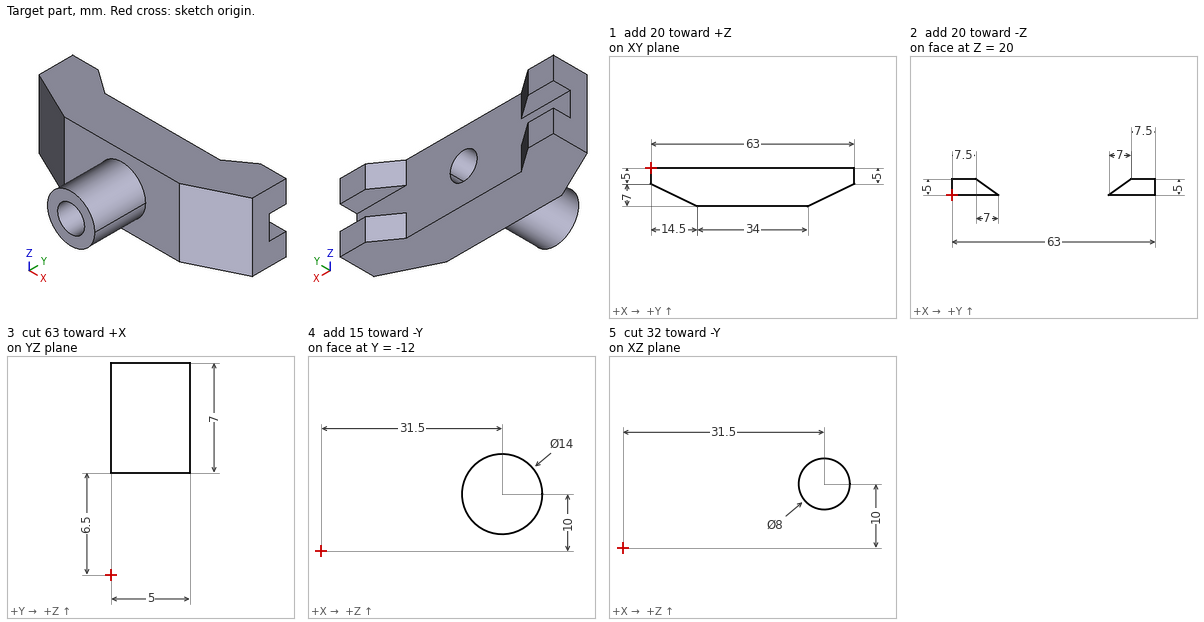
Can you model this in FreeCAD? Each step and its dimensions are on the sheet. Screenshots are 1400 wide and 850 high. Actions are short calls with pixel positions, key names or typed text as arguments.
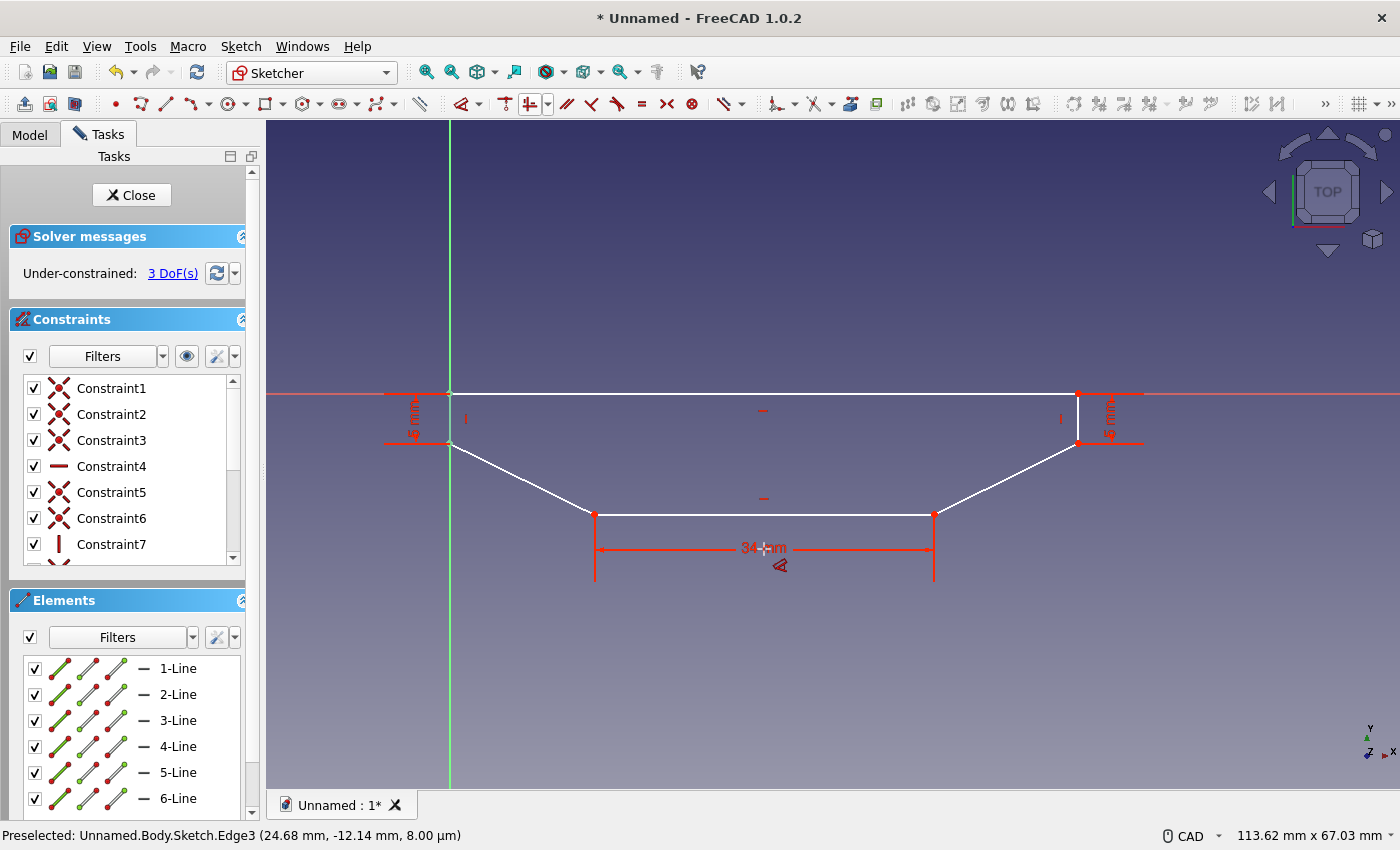
click(890, 394)
click(764, 360)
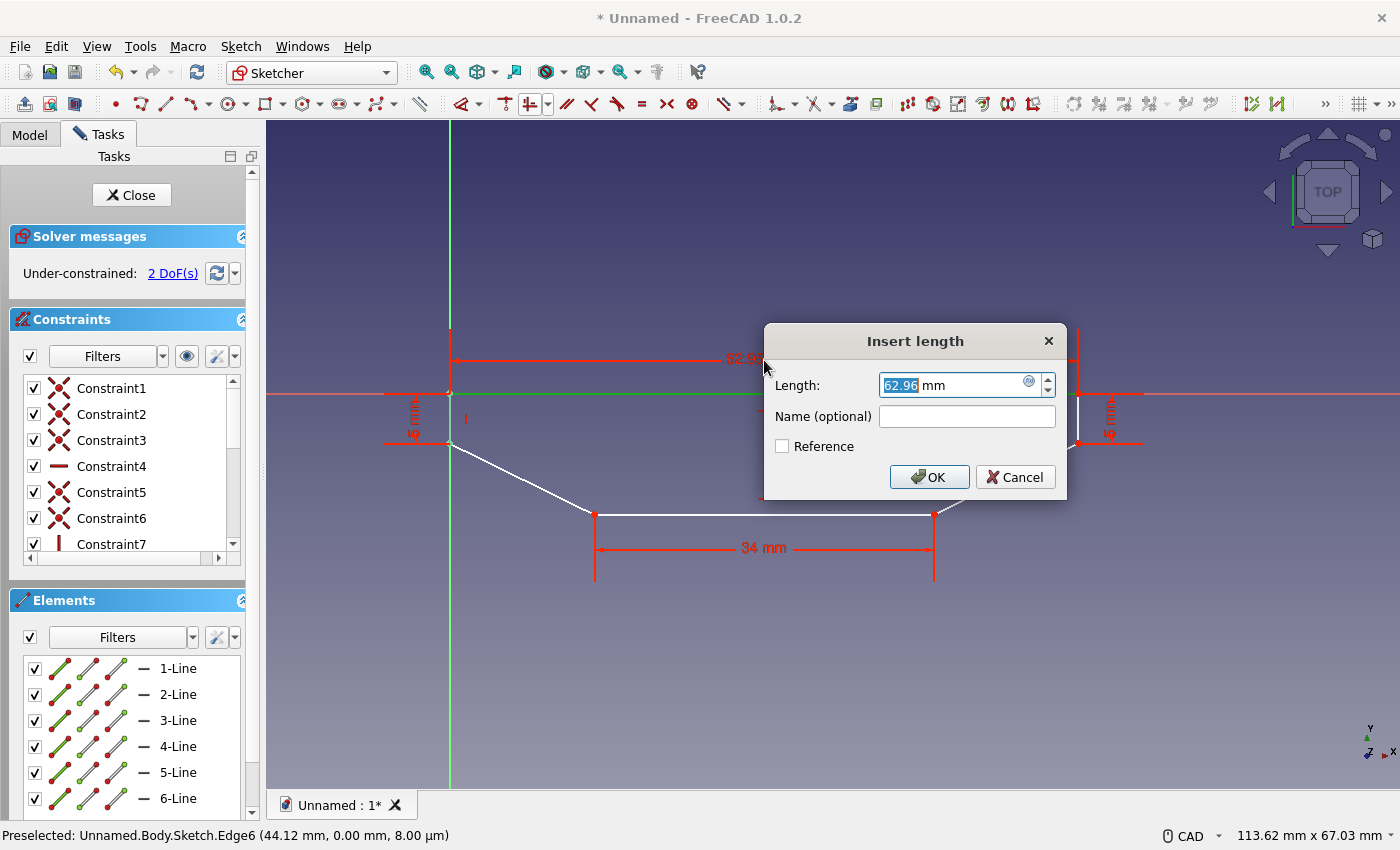
text(63)
key(Return)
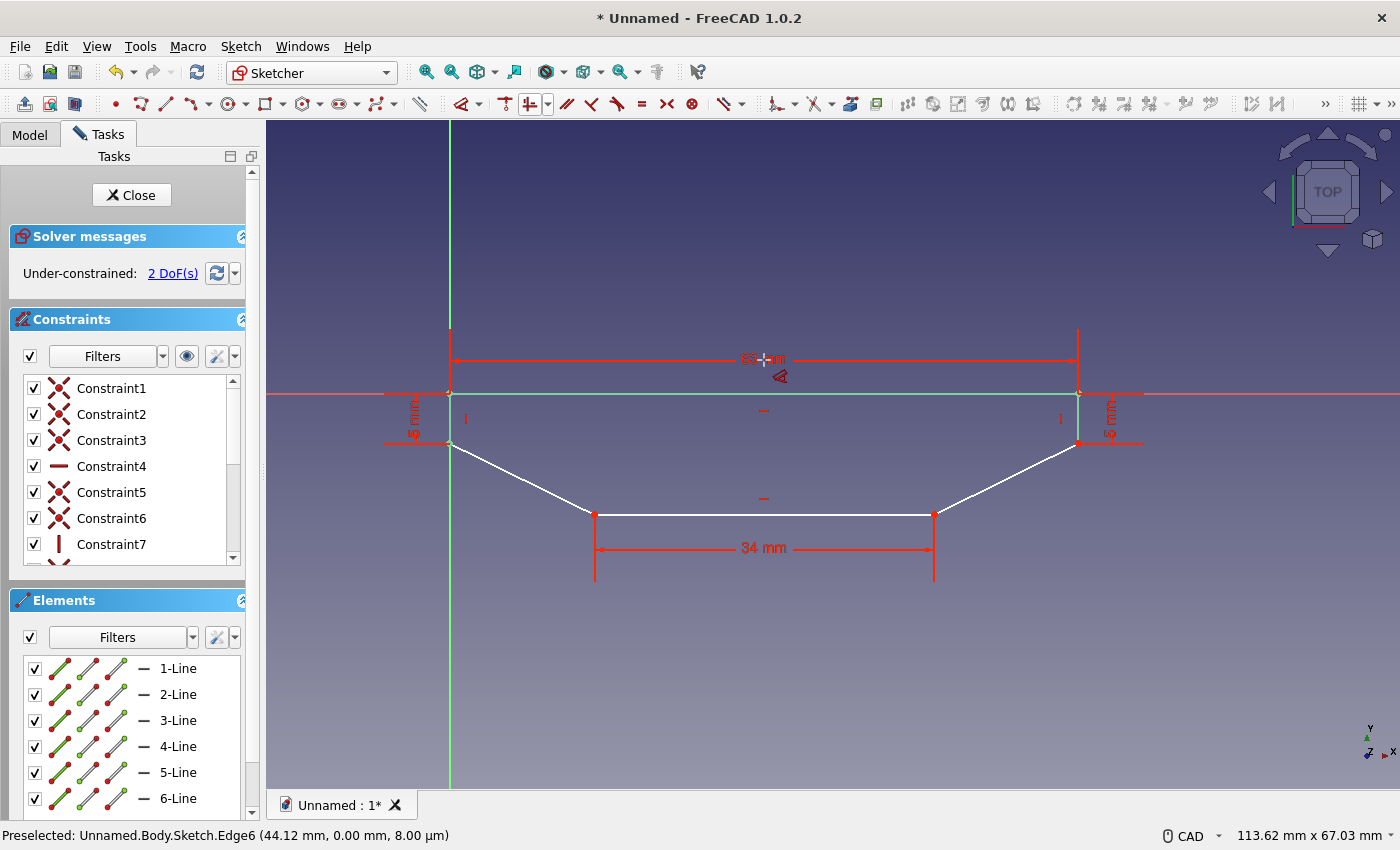
click(493, 465)
click(416, 479)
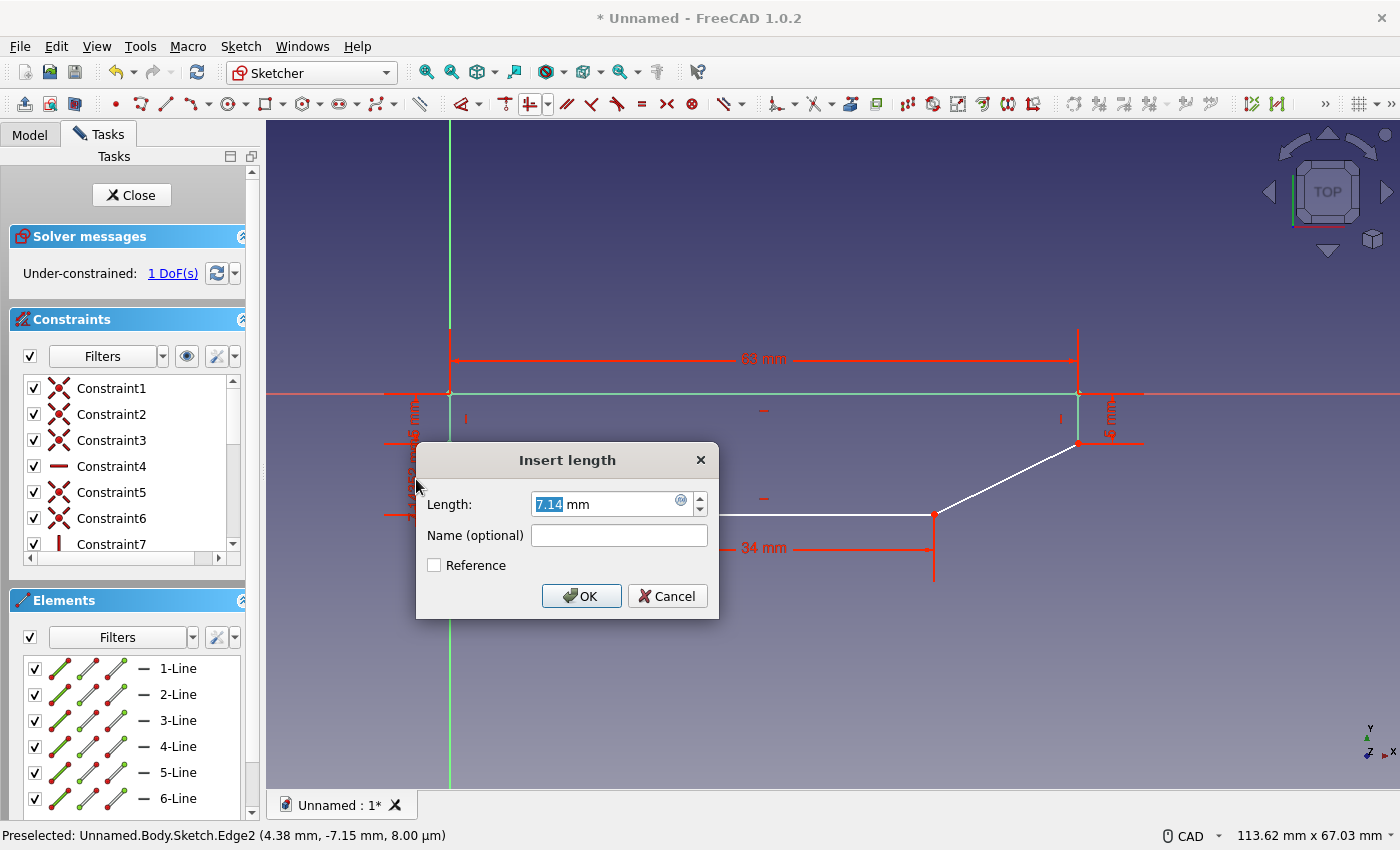
text(7)
key(Return)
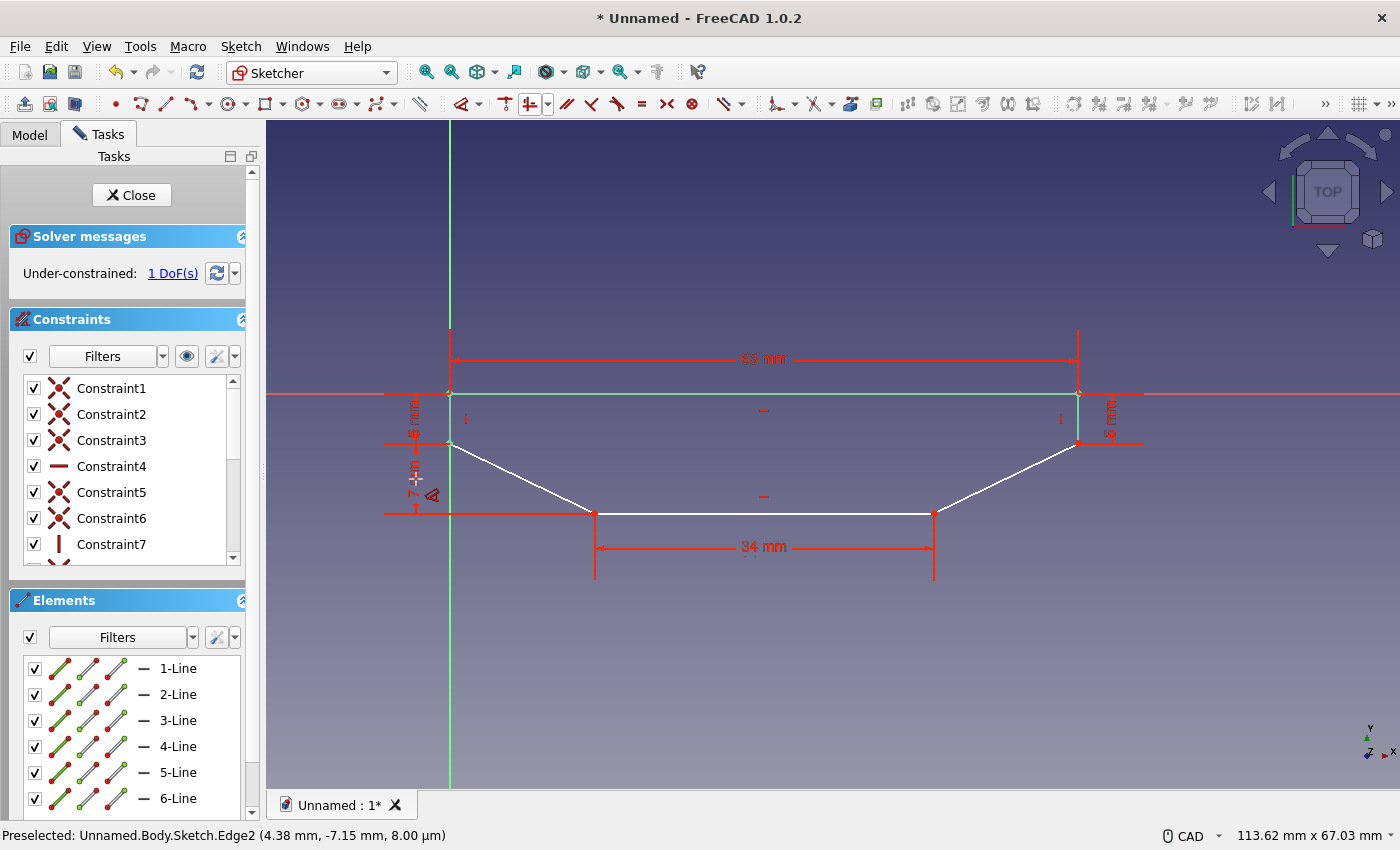
click(595, 514)
click(522, 548)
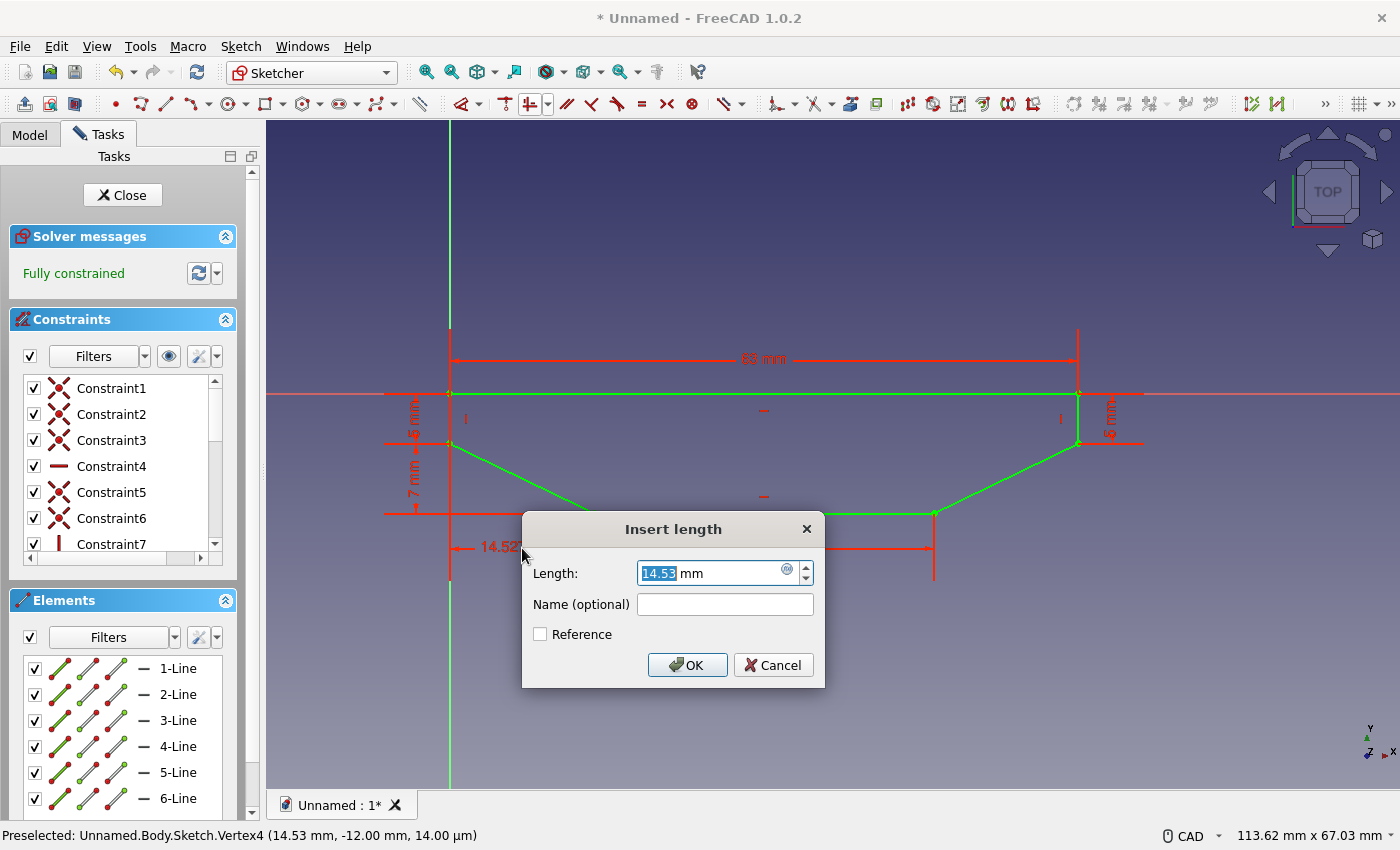
text(14.5)
key(Return)
key(Escape)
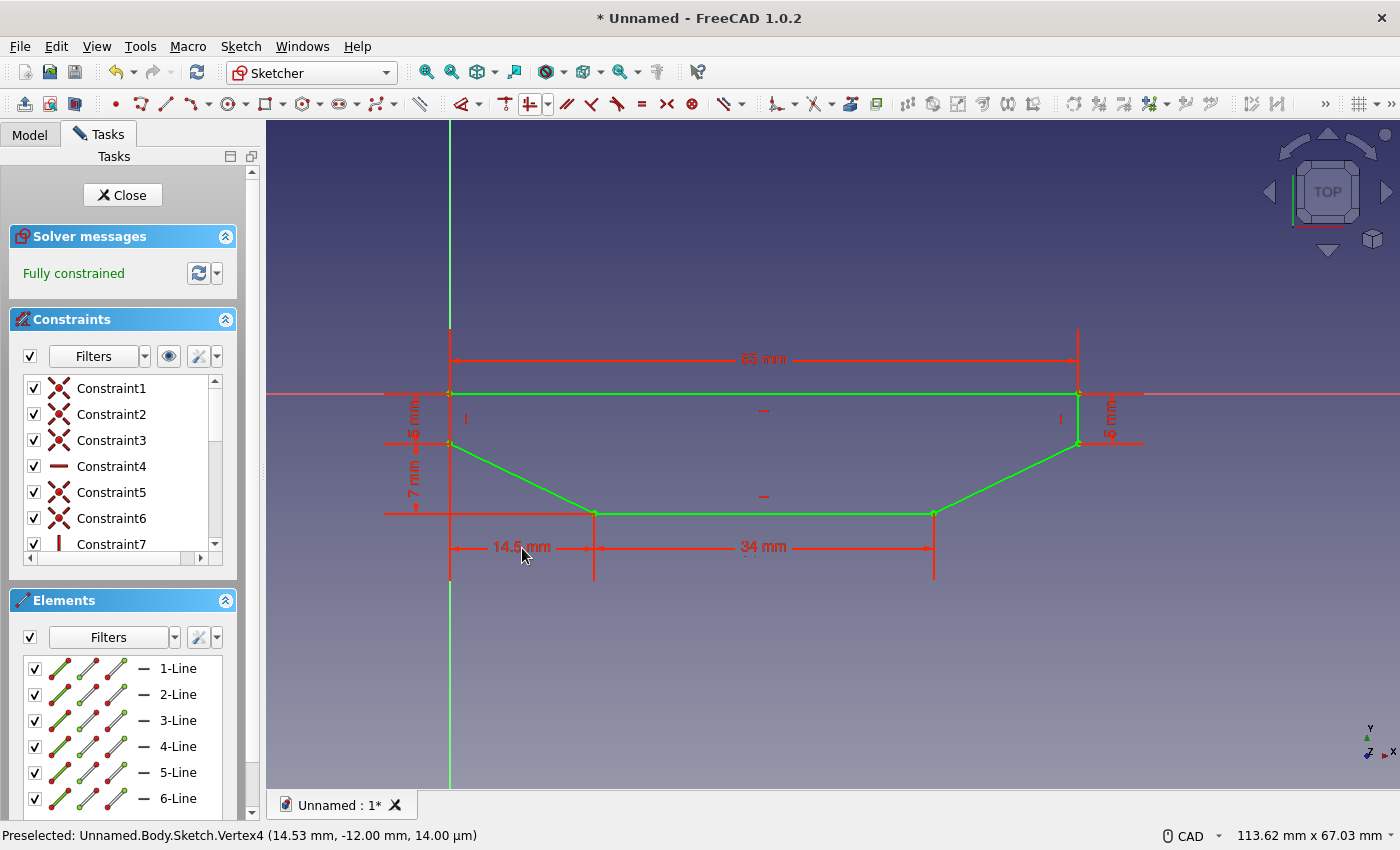
click(123, 195)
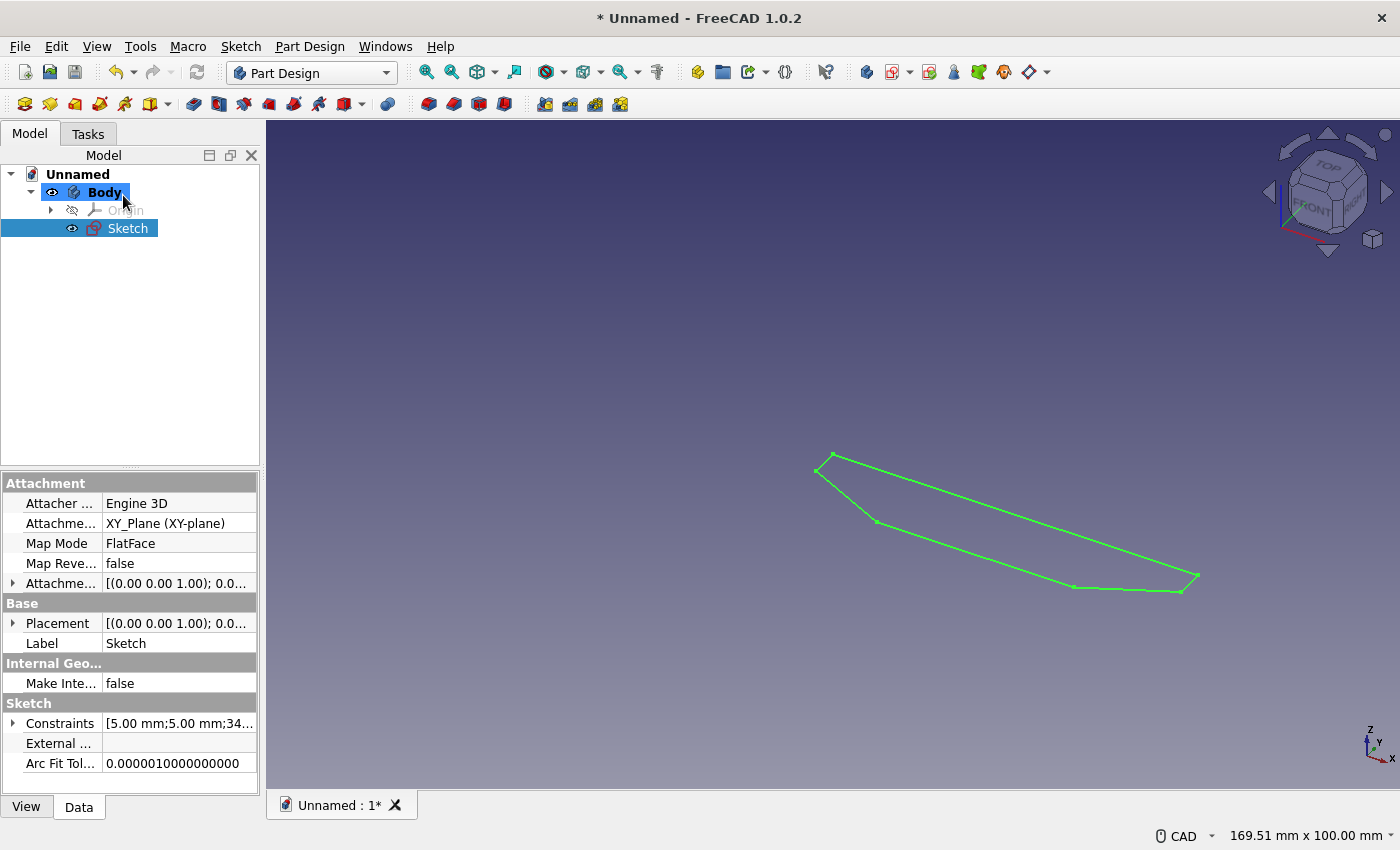
click(25, 104)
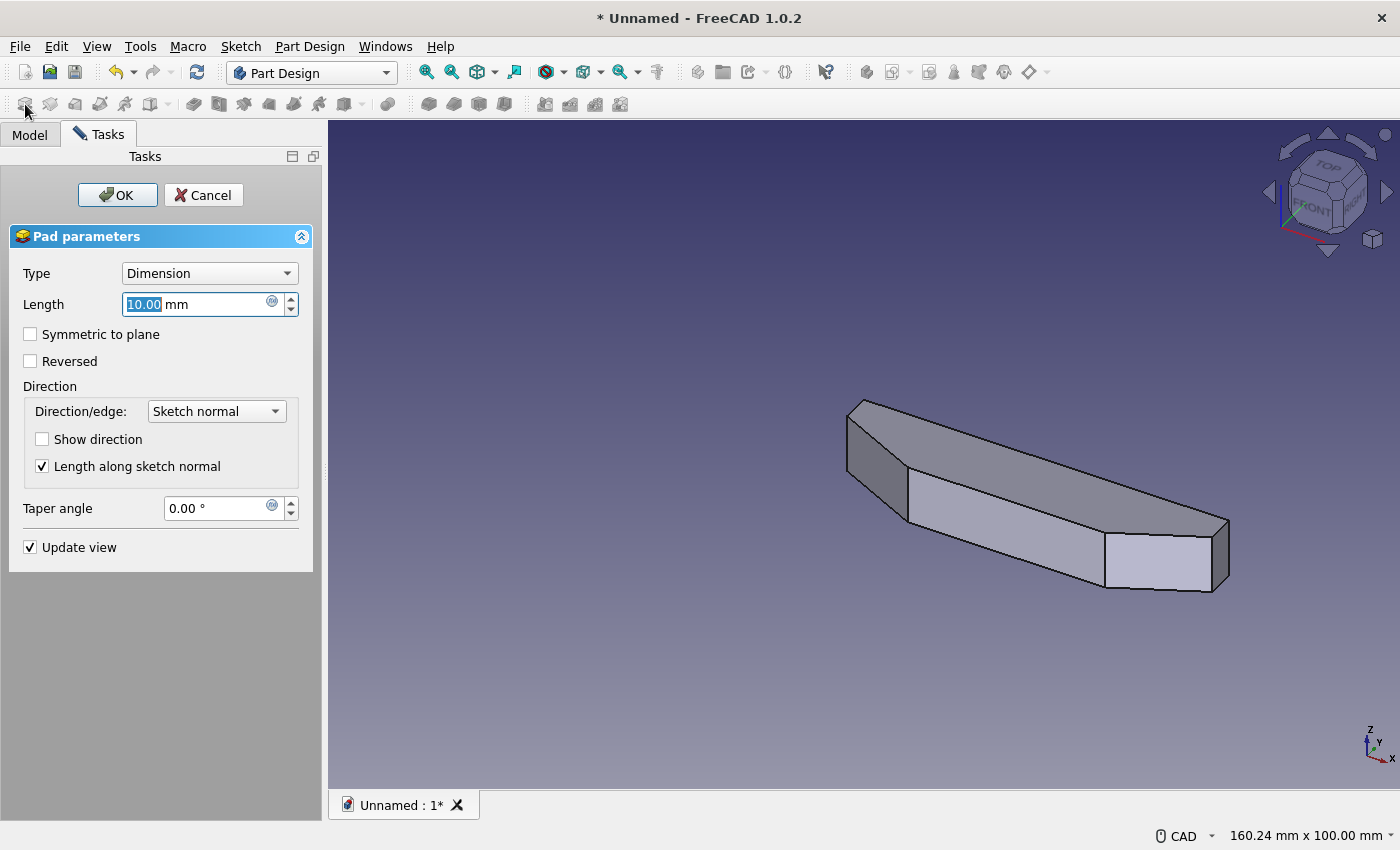
text(20)
key(Tab)